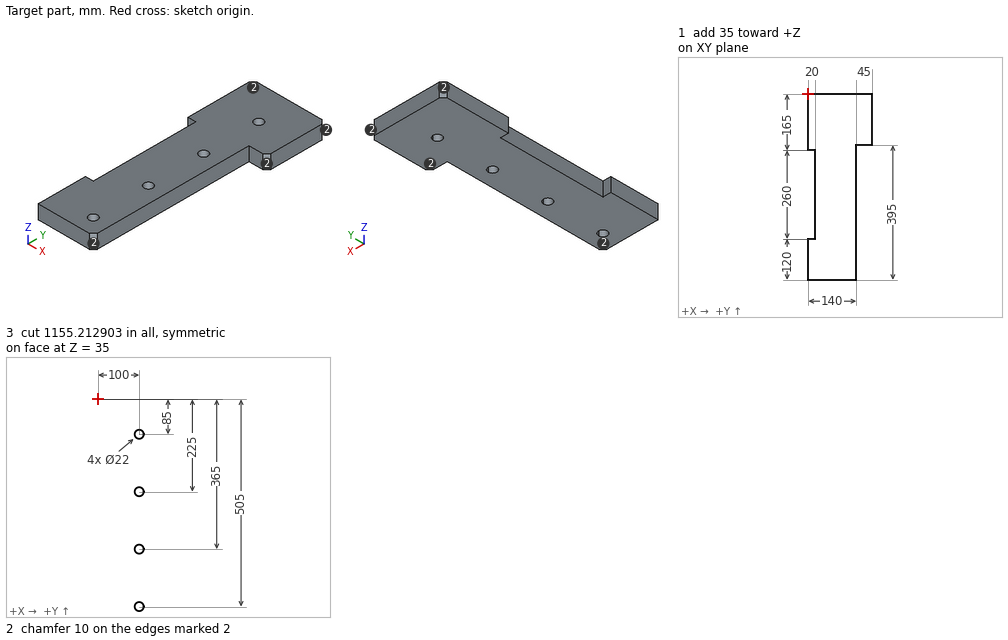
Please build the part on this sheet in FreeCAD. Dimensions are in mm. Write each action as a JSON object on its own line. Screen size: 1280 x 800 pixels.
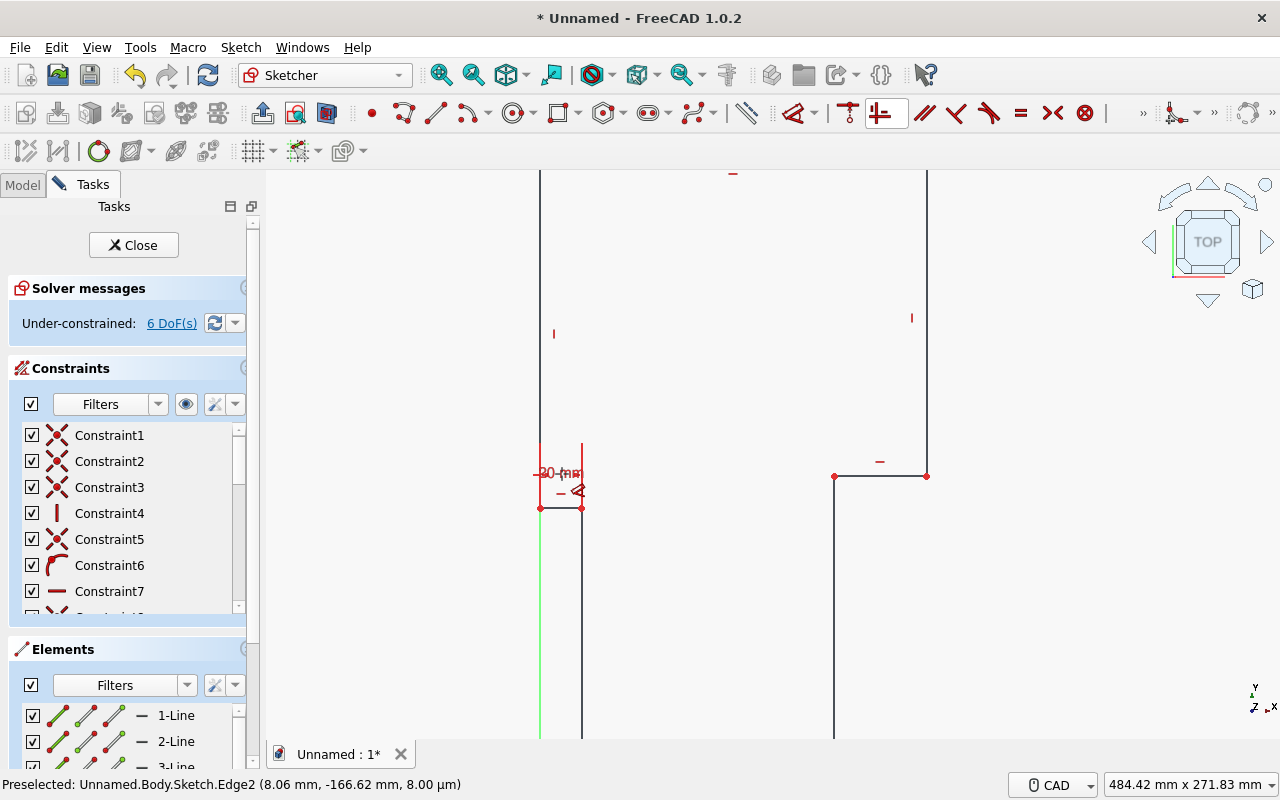
{"action": "left_click", "coordinate": [862, 476]}
{"action": "left_click", "coordinate": [880, 442]}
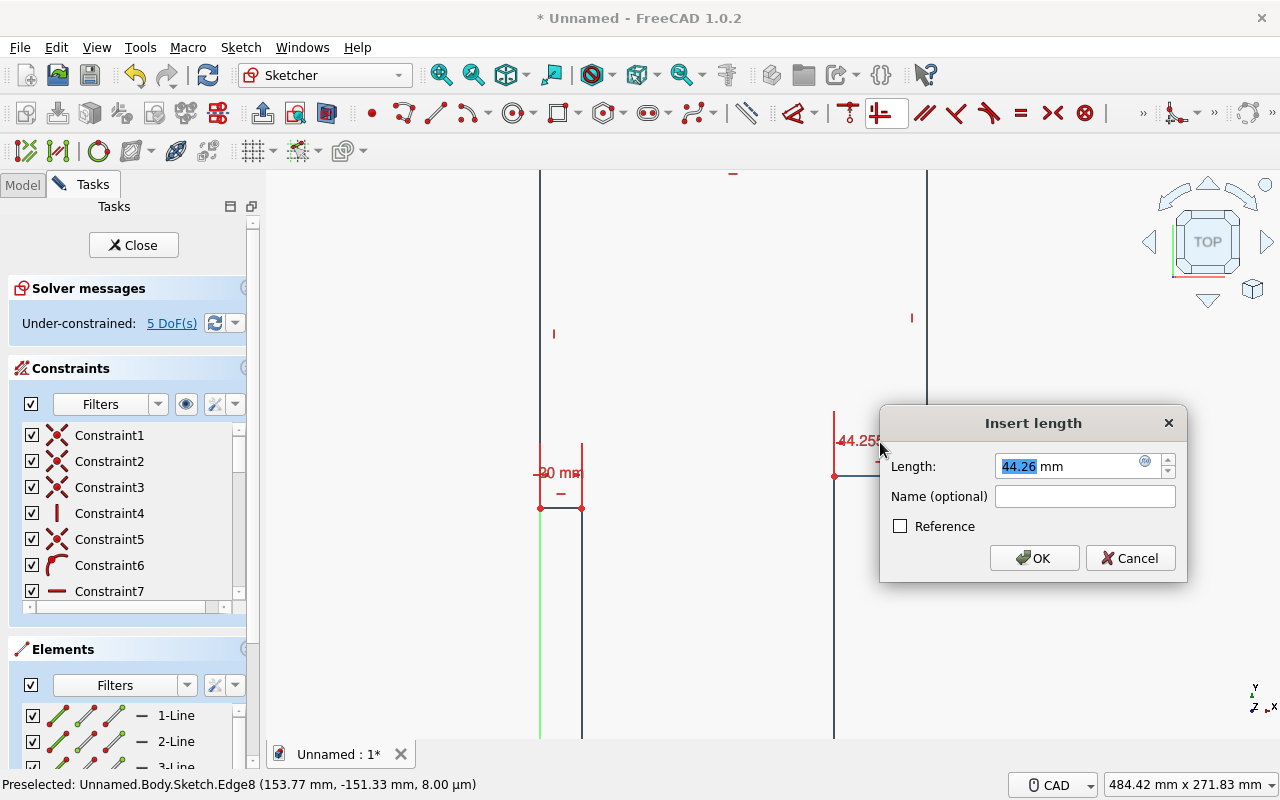
{"action": "type", "text": "45"}
{"action": "key", "text": "Return"}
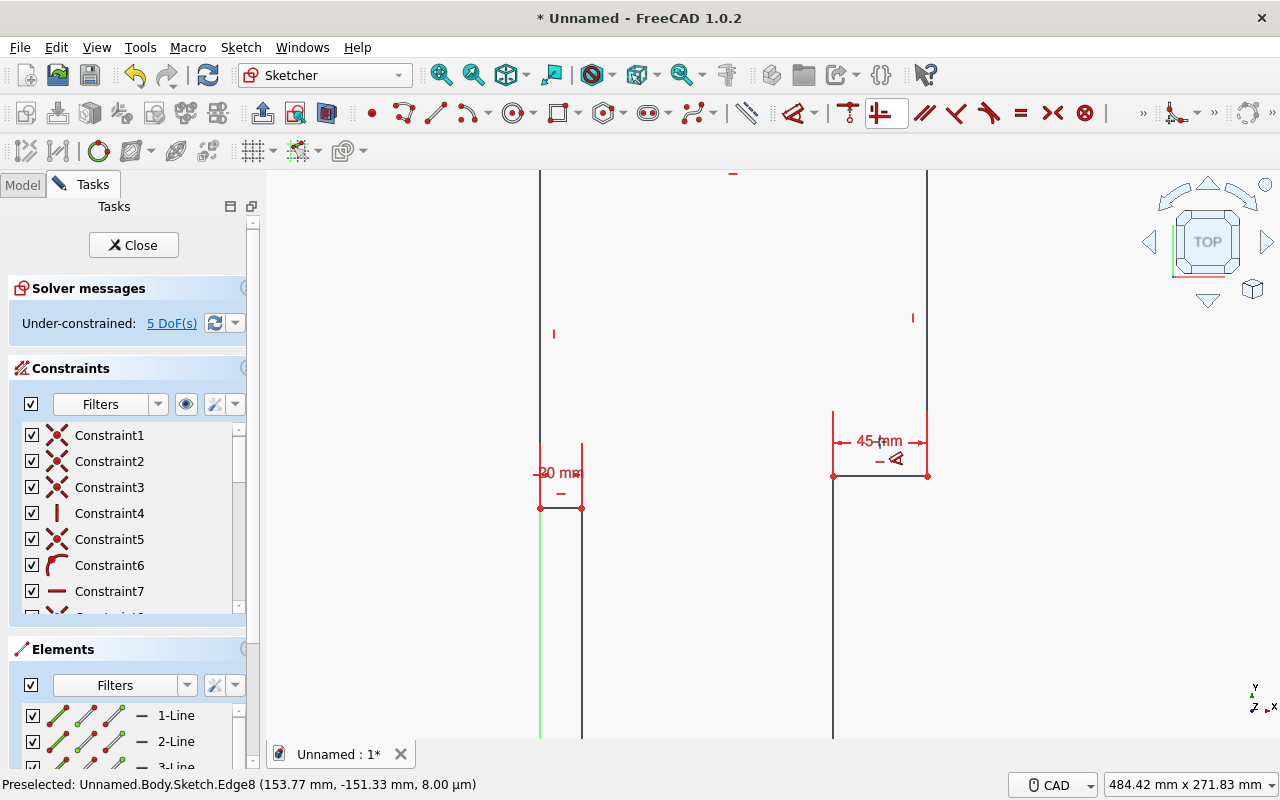
{"action": "left_click", "coordinate": [540, 264]}
{"action": "left_click", "coordinate": [506, 353]}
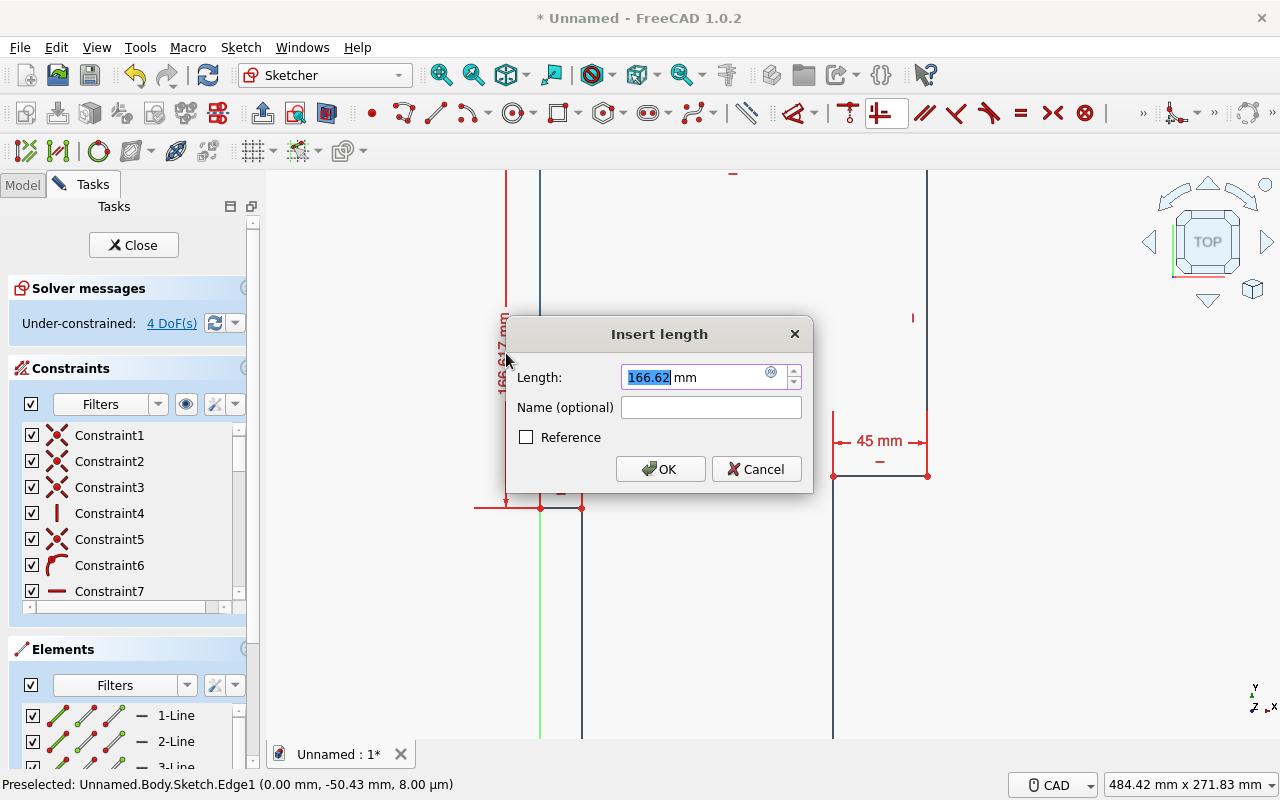
{"action": "type", "text": "165"}
{"action": "key", "text": "Return"}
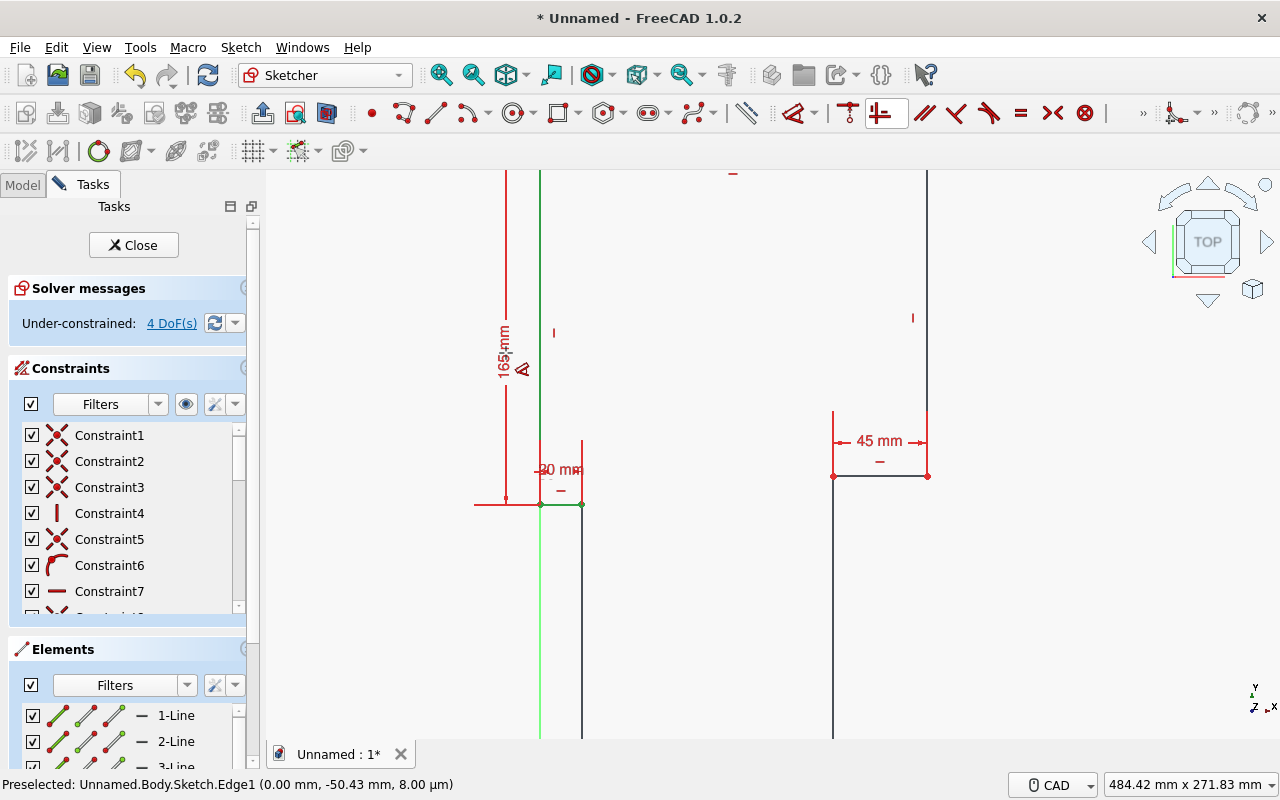
{"action": "left_click", "coordinate": [582, 669]}
{"action": "left_click", "coordinate": [616, 608]}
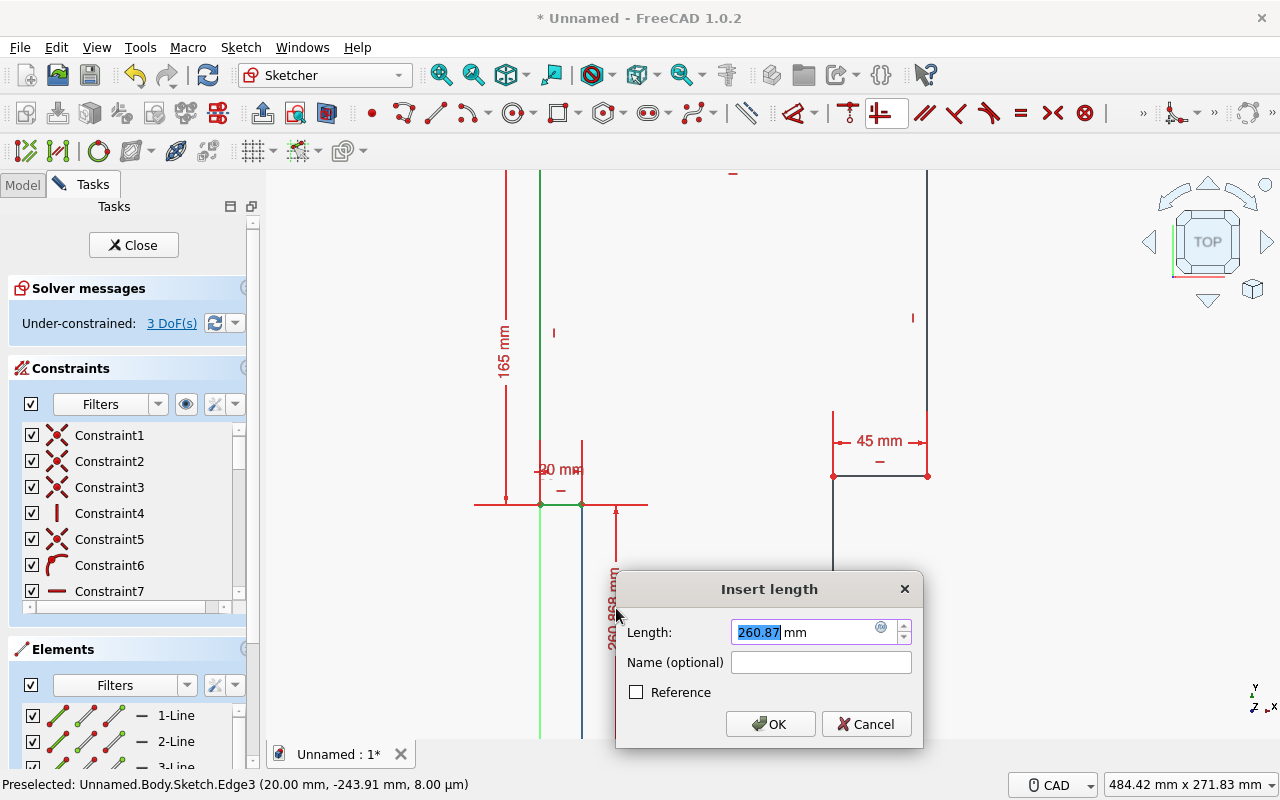
{"action": "type", "text": "260"}
{"action": "key", "text": "Return"}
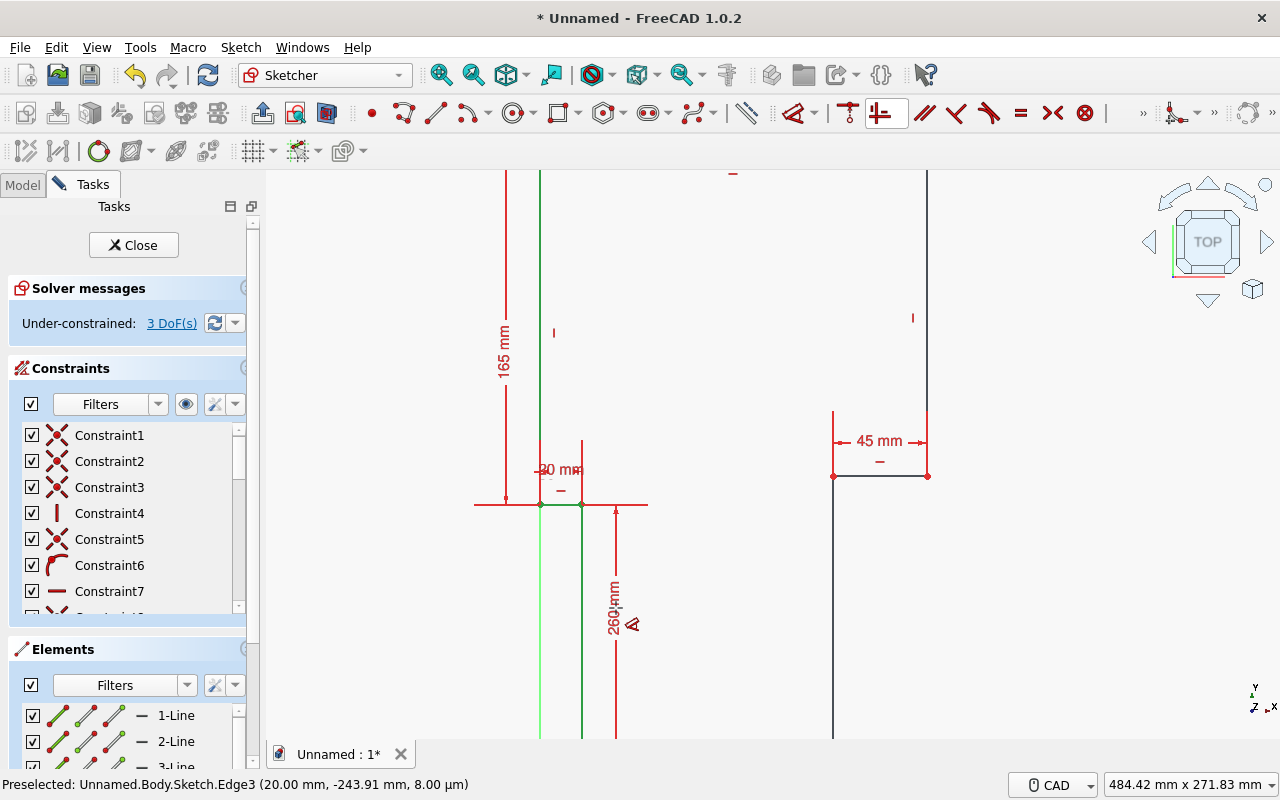
{"action": "scroll", "coordinate": [692, 336], "scroll_direction": "down", "scroll_amount": 6}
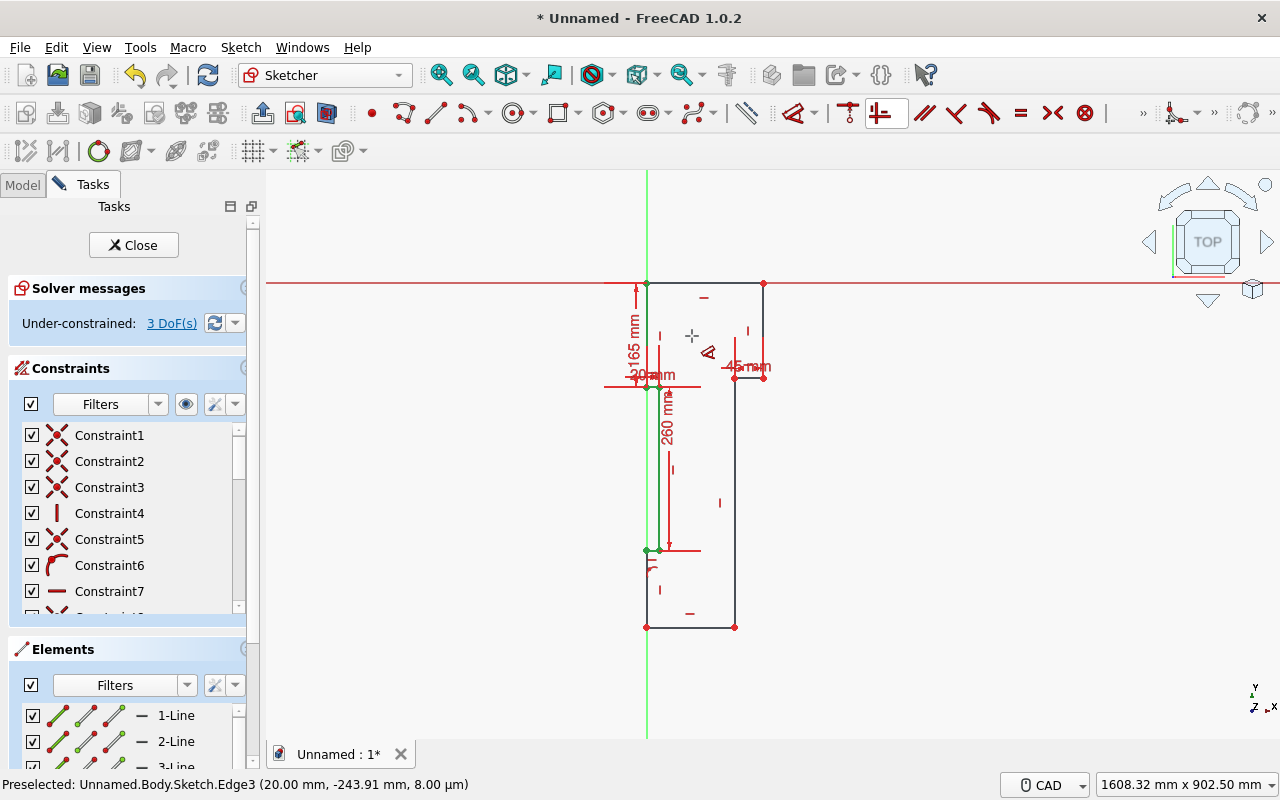
{"action": "left_click", "coordinate": [647, 574]}
{"action": "left_click", "coordinate": [613, 589]}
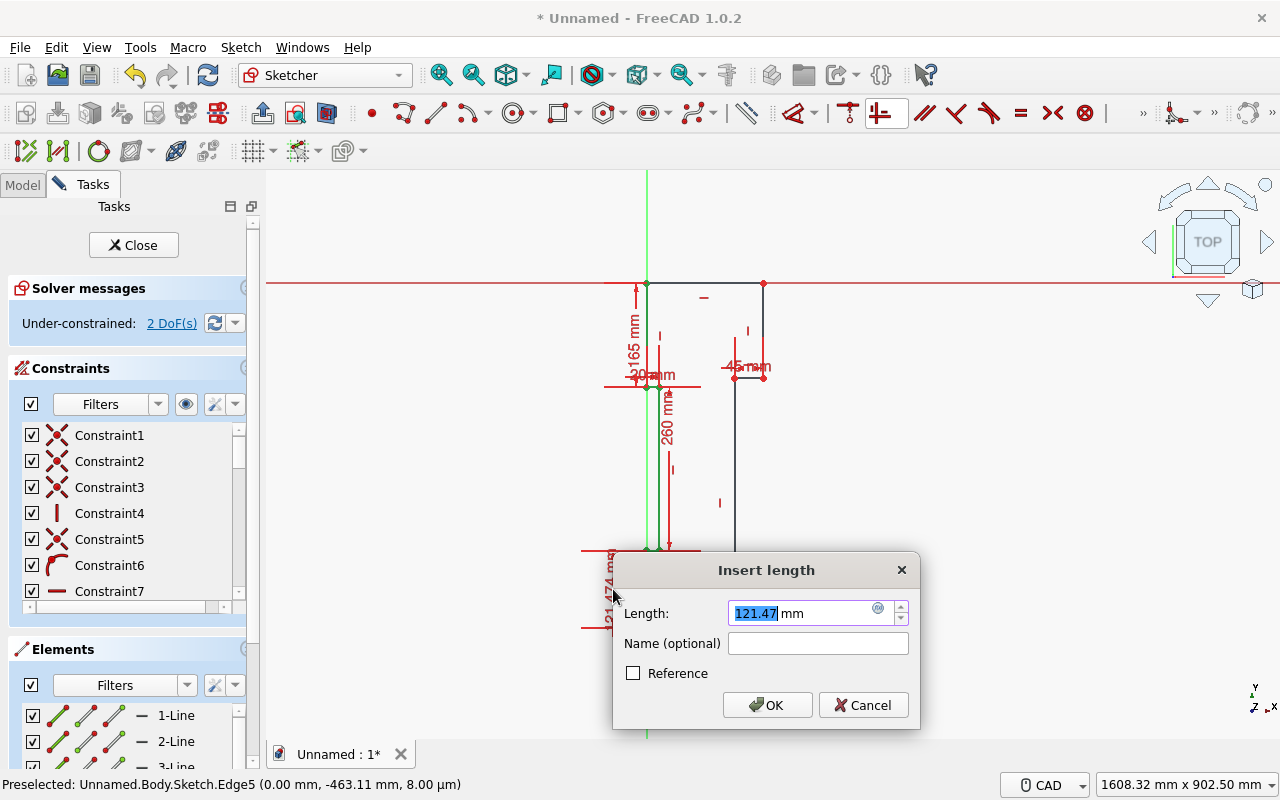
{"action": "type", "text": "120"}
{"action": "key", "text": "Return"}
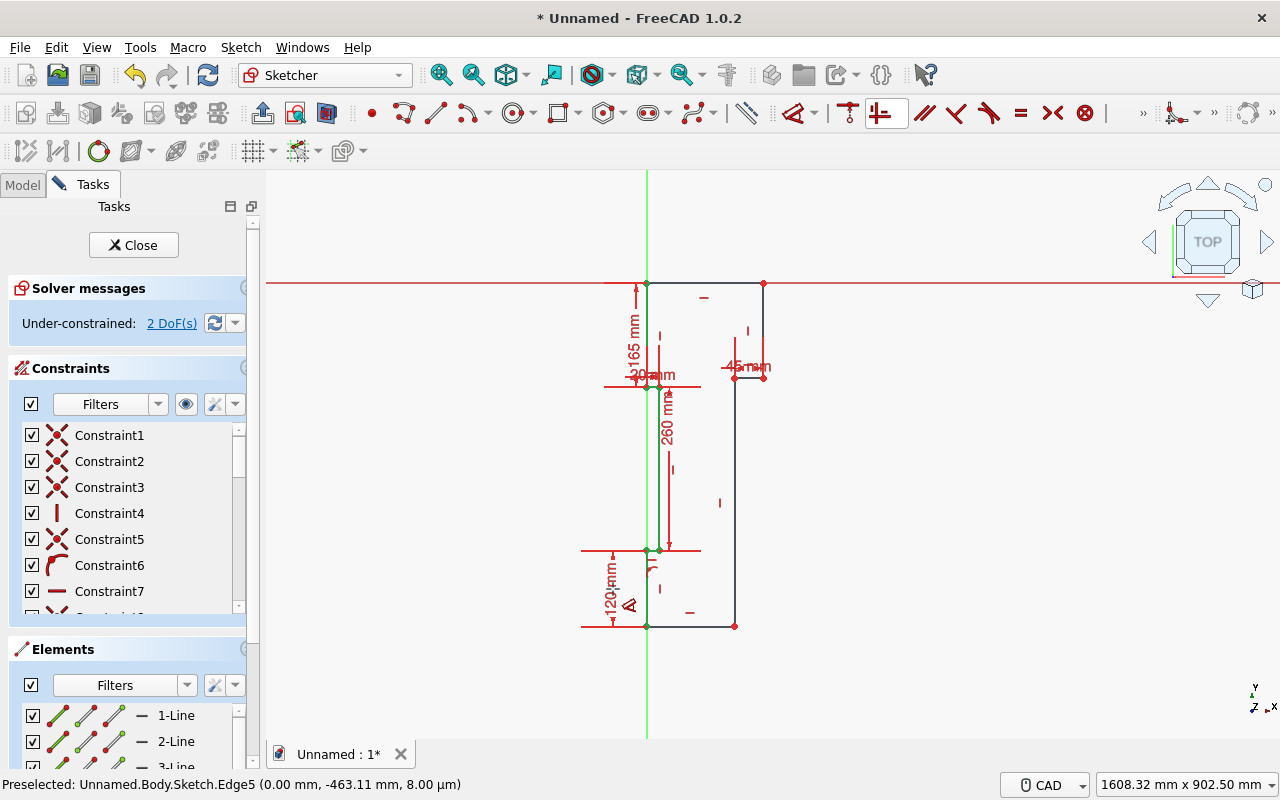
{"action": "left_click", "coordinate": [673, 627]}
{"action": "left_click", "coordinate": [691, 661]}